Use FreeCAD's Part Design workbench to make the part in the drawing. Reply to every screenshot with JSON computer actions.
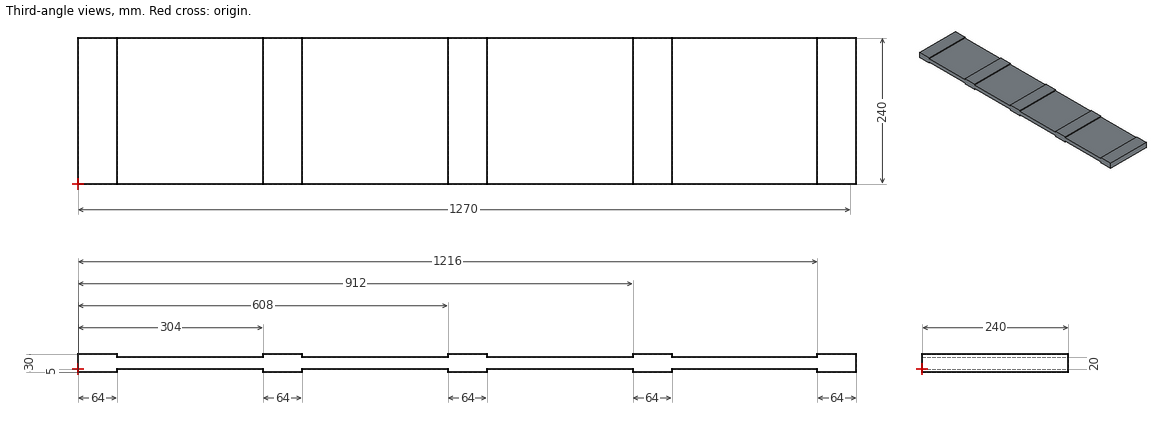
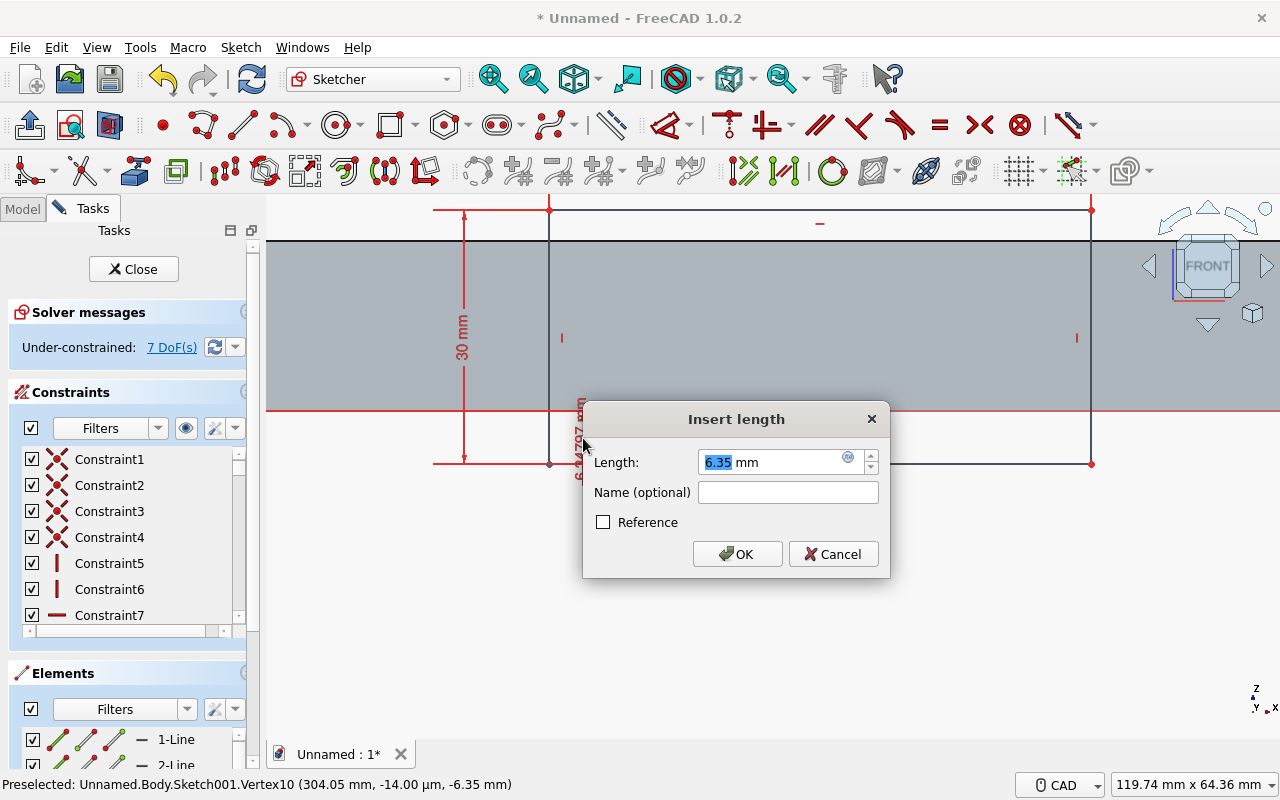
{"action": "type", "text": "5"}
{"action": "key", "text": "Return"}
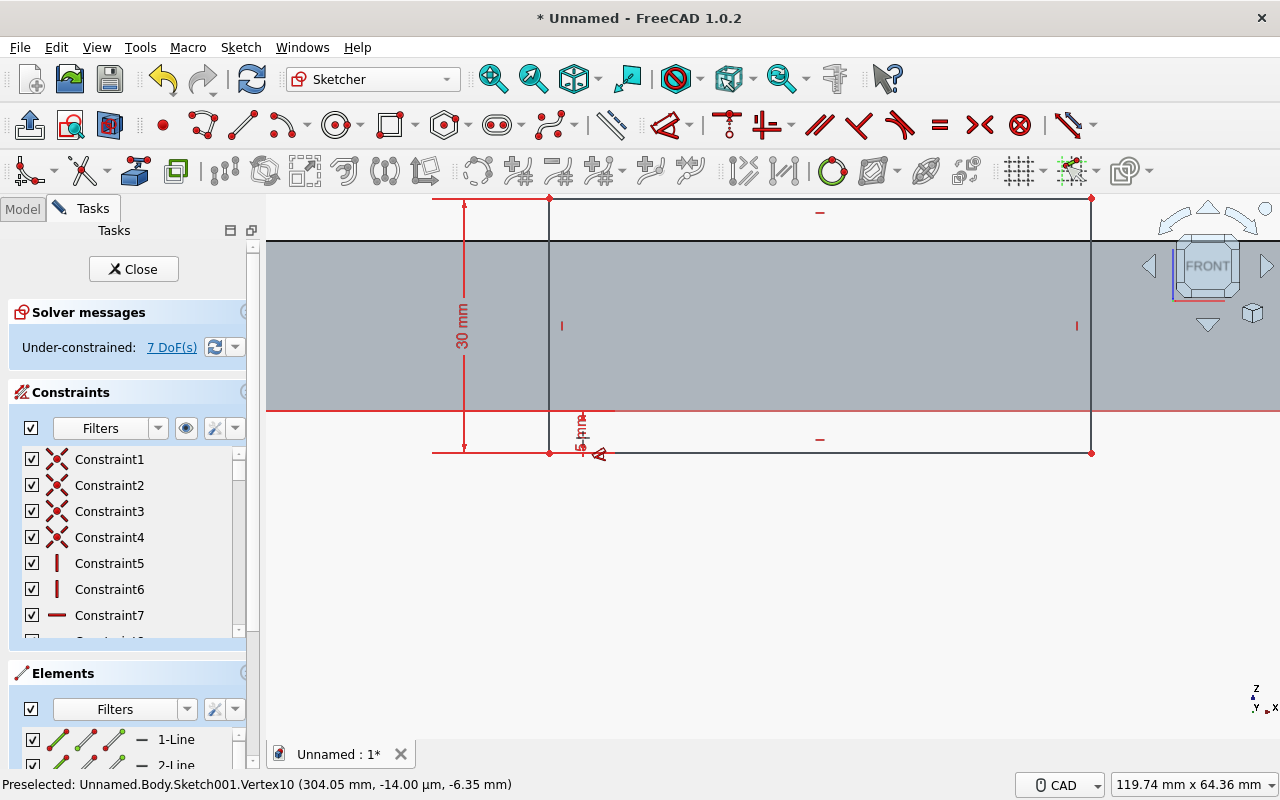
{"action": "scroll", "coordinate": [564, 474], "scroll_direction": "down", "scroll_amount": 15}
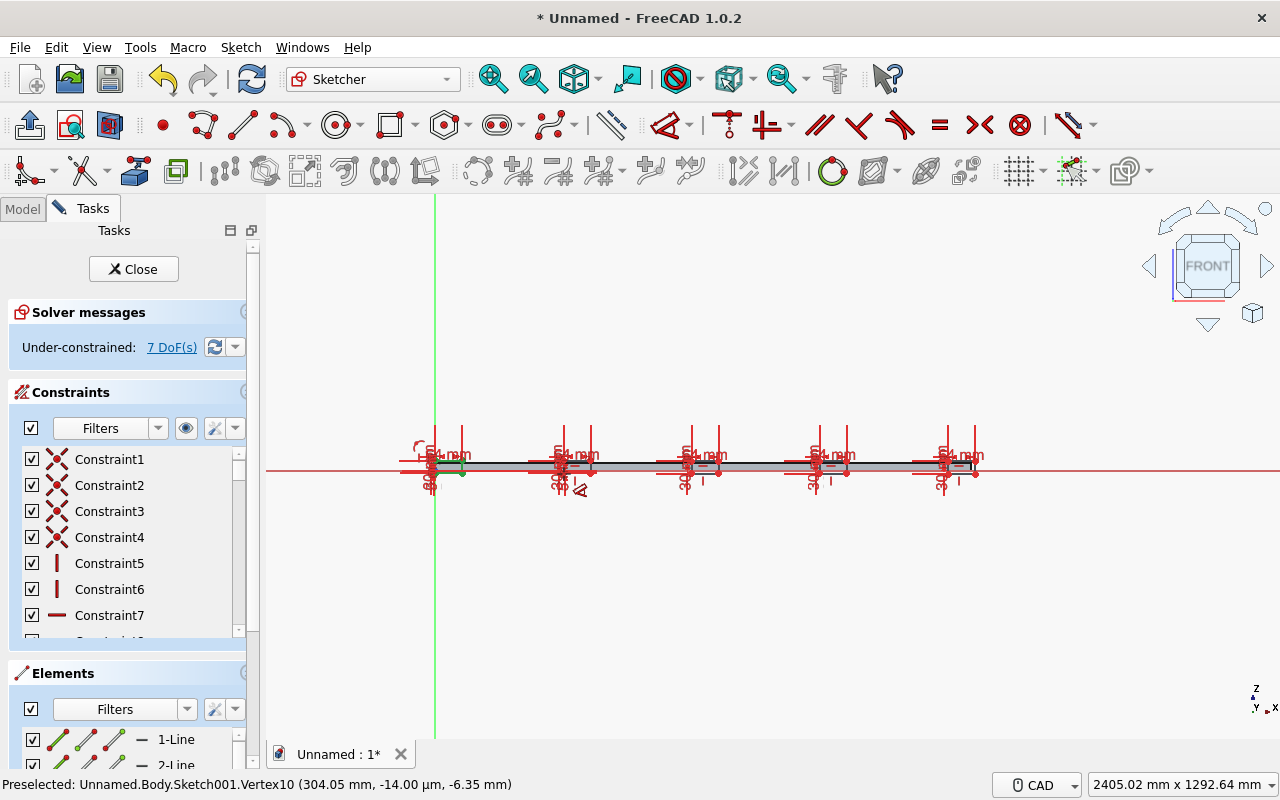
{"action": "scroll", "coordinate": [692, 474], "scroll_direction": "up", "scroll_amount": 15}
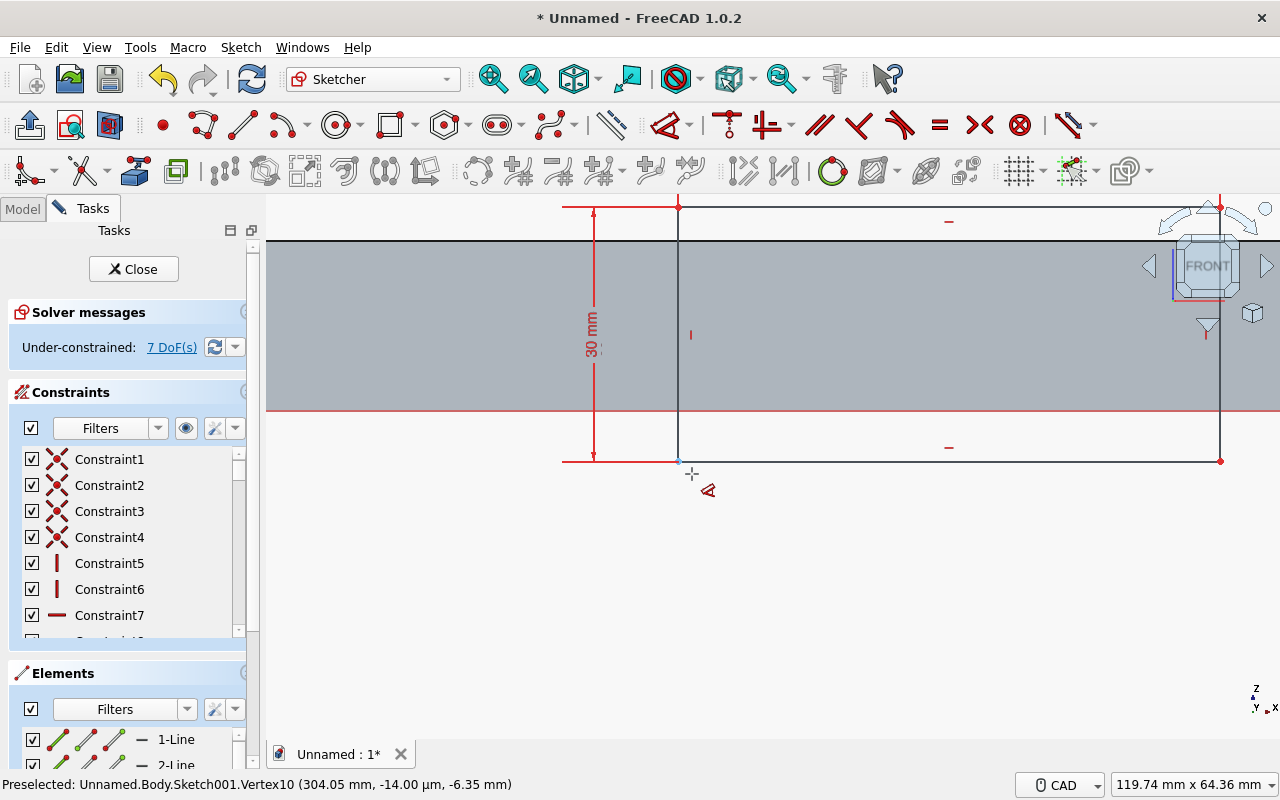
{"action": "left_click", "coordinate": [678, 462]}
{"action": "left_click", "coordinate": [712, 436]}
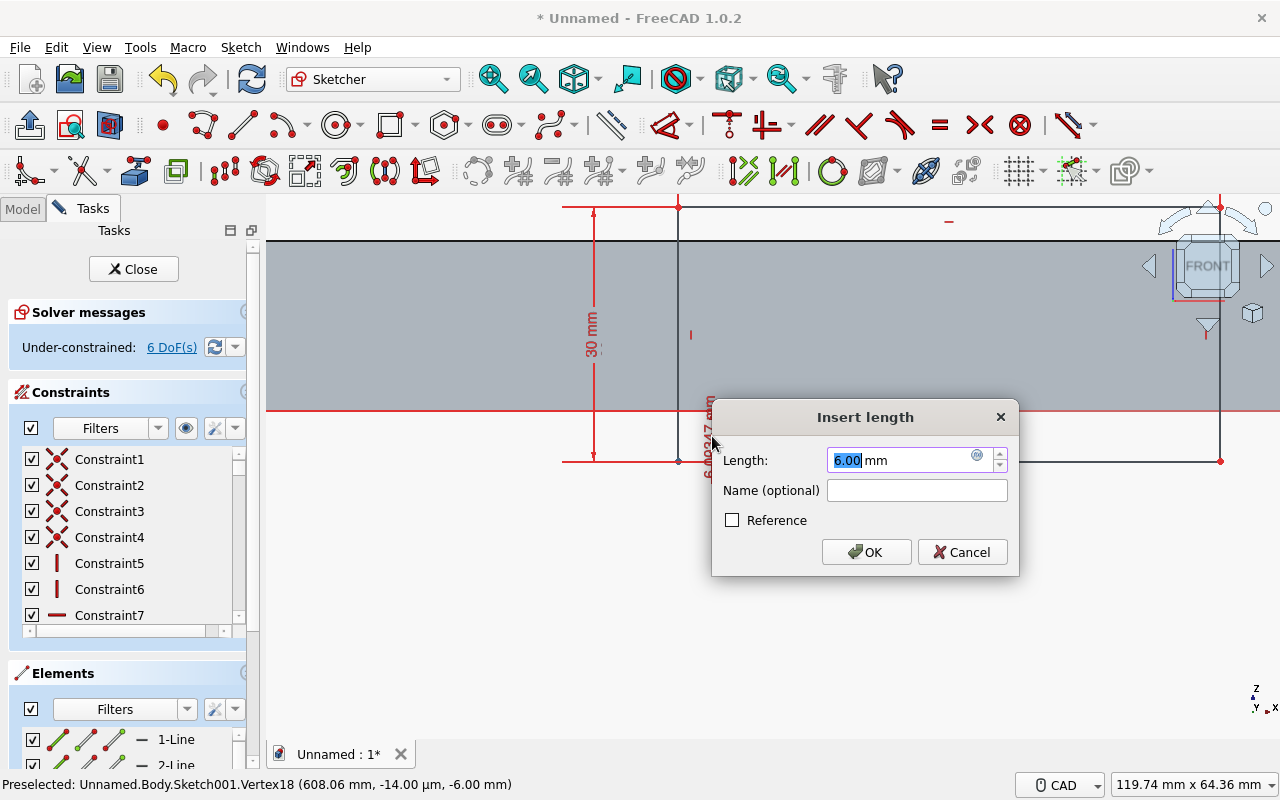
{"action": "type", "text": "5"}
{"action": "key", "text": "Return"}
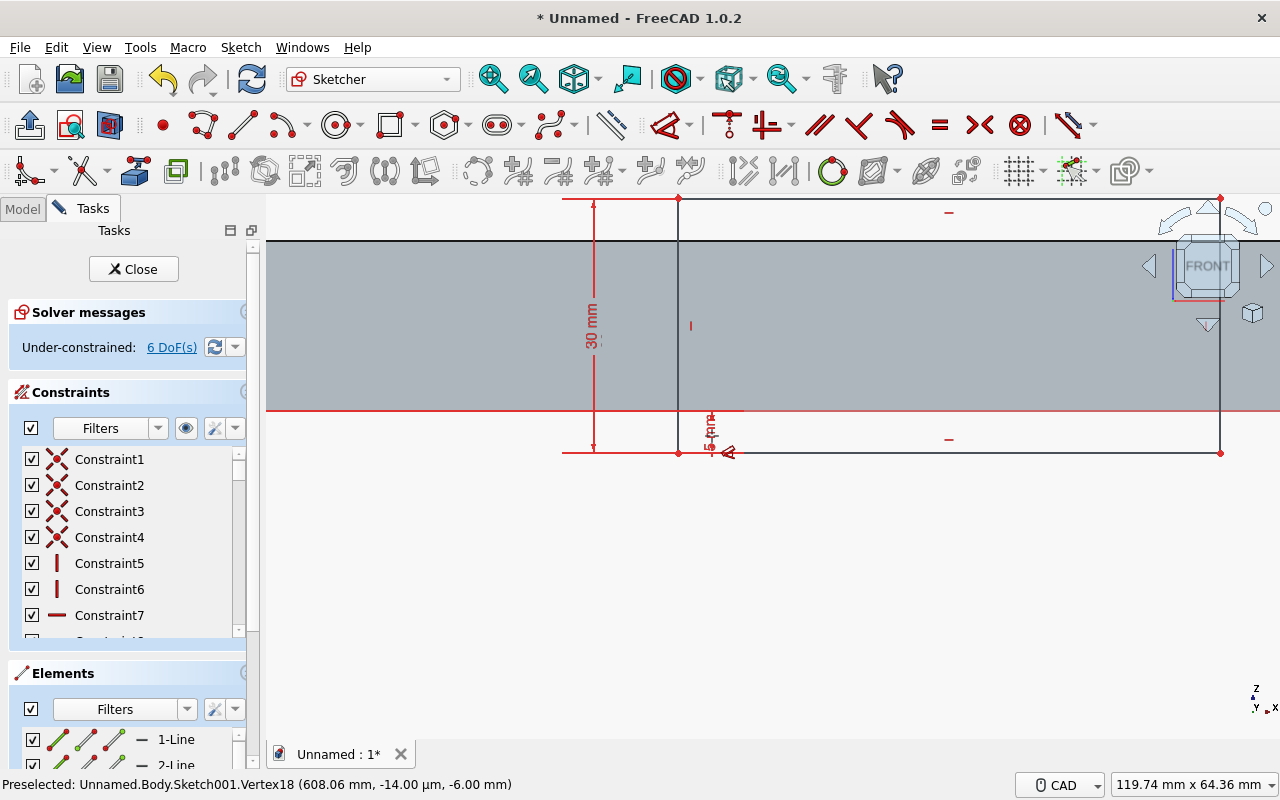
{"action": "scroll", "coordinate": [692, 474], "scroll_direction": "down", "scroll_amount": 15}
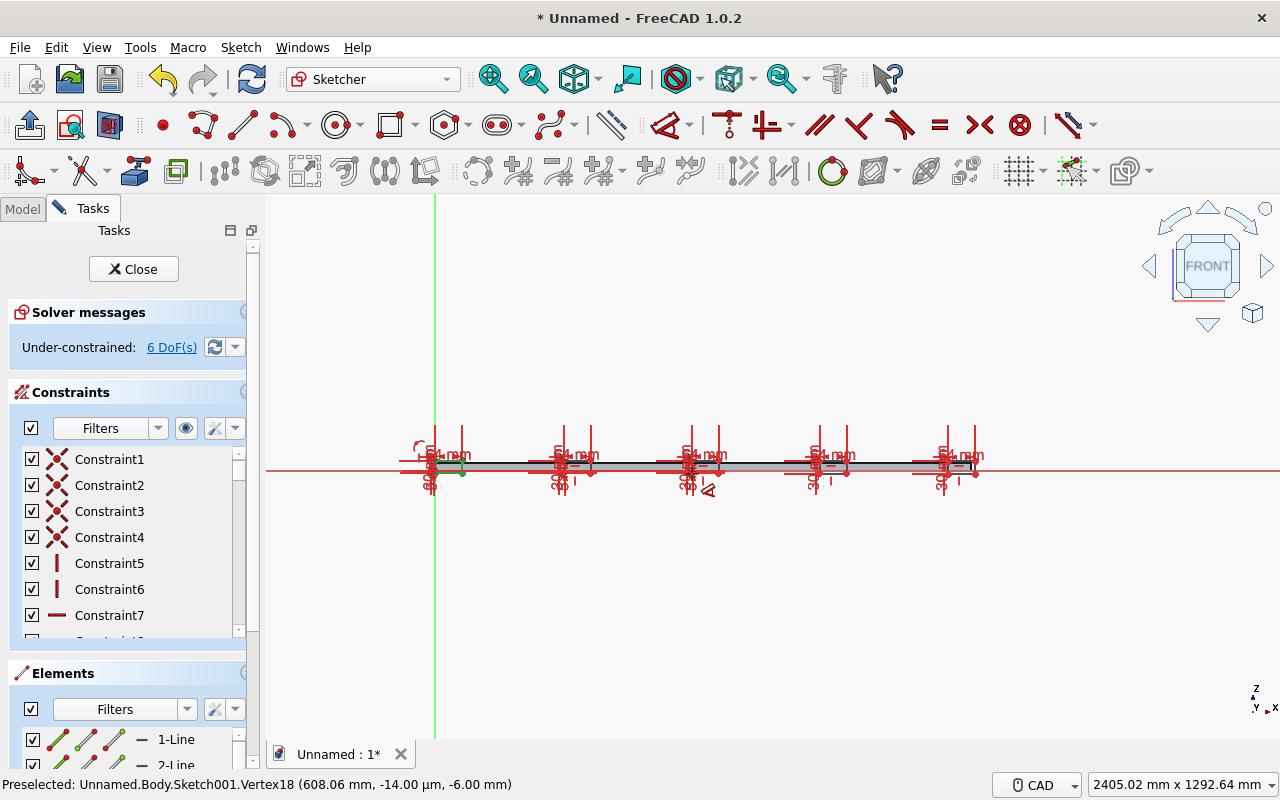
{"action": "scroll", "coordinate": [820, 474], "scroll_direction": "up", "scroll_amount": 15}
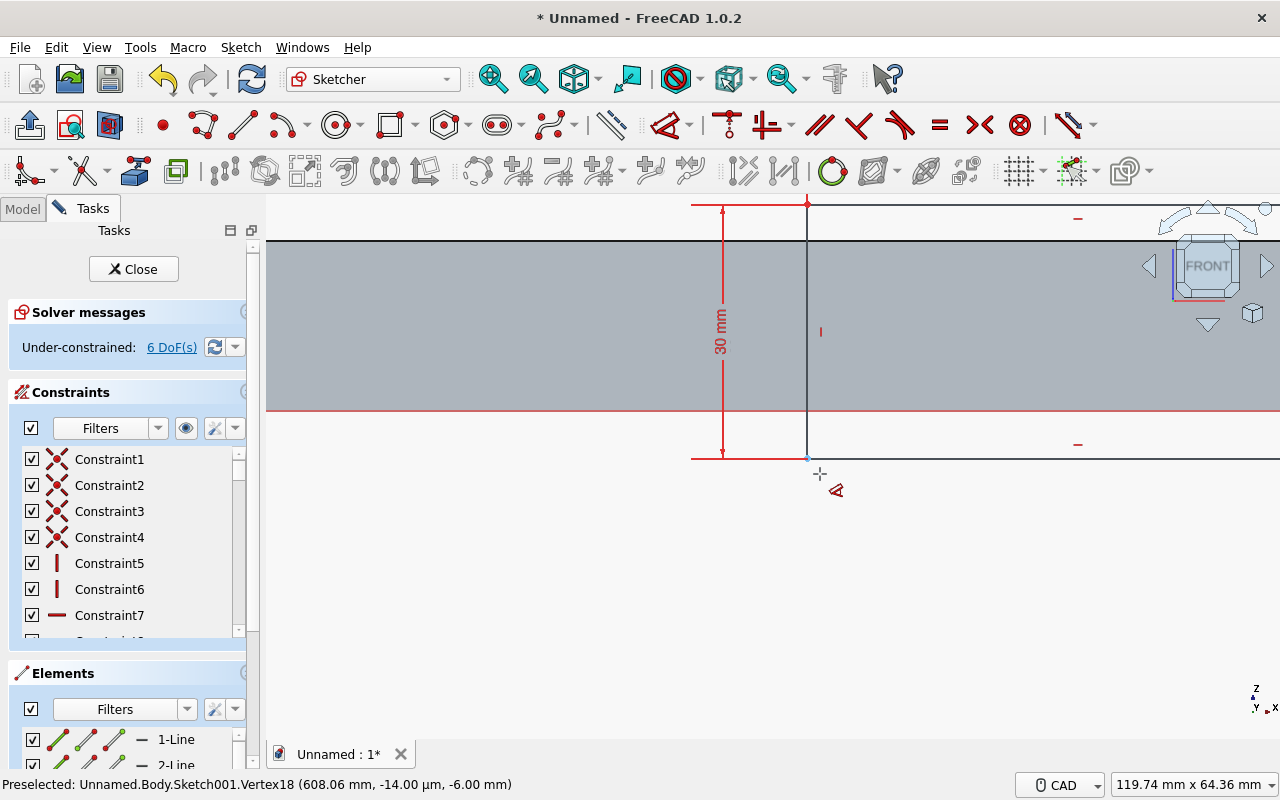
{"action": "left_click", "coordinate": [807, 459]}
{"action": "left_click", "coordinate": [841, 435]}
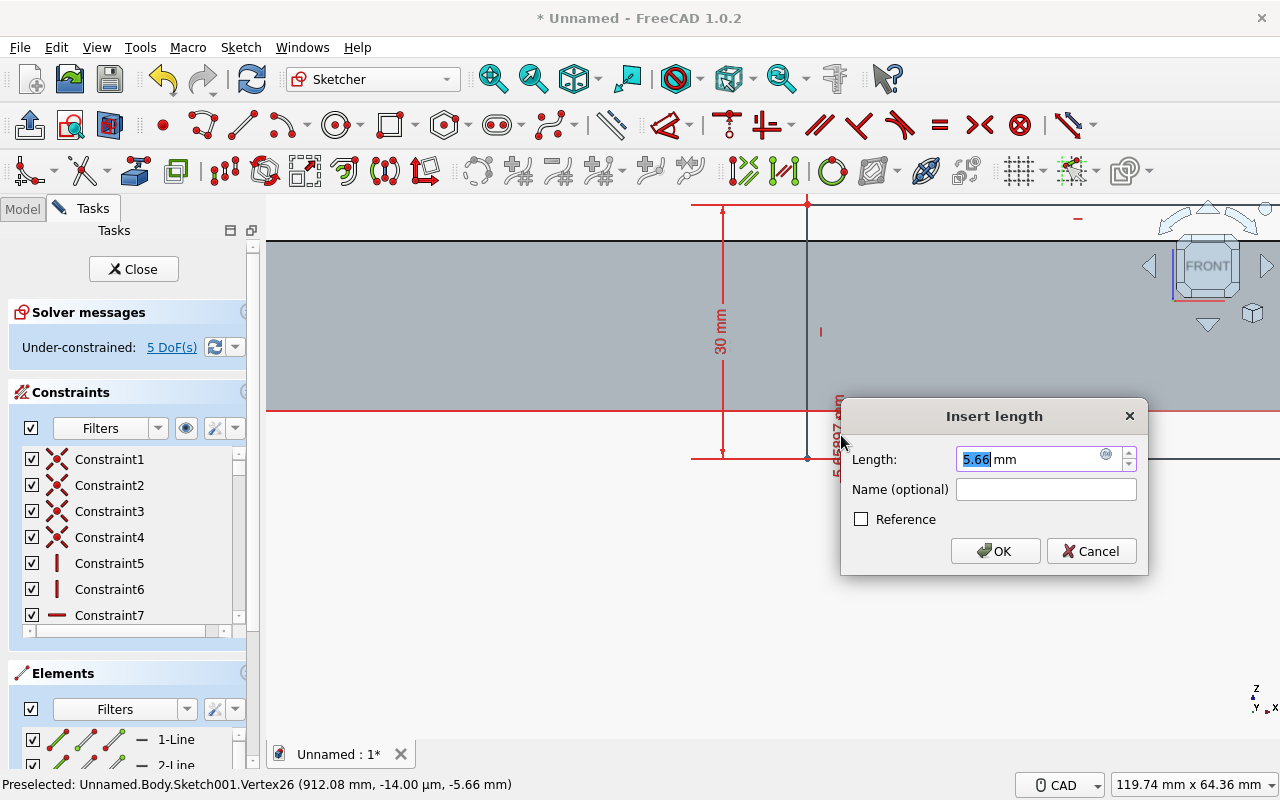
{"action": "type", "text": "5"}
{"action": "key", "text": "Return"}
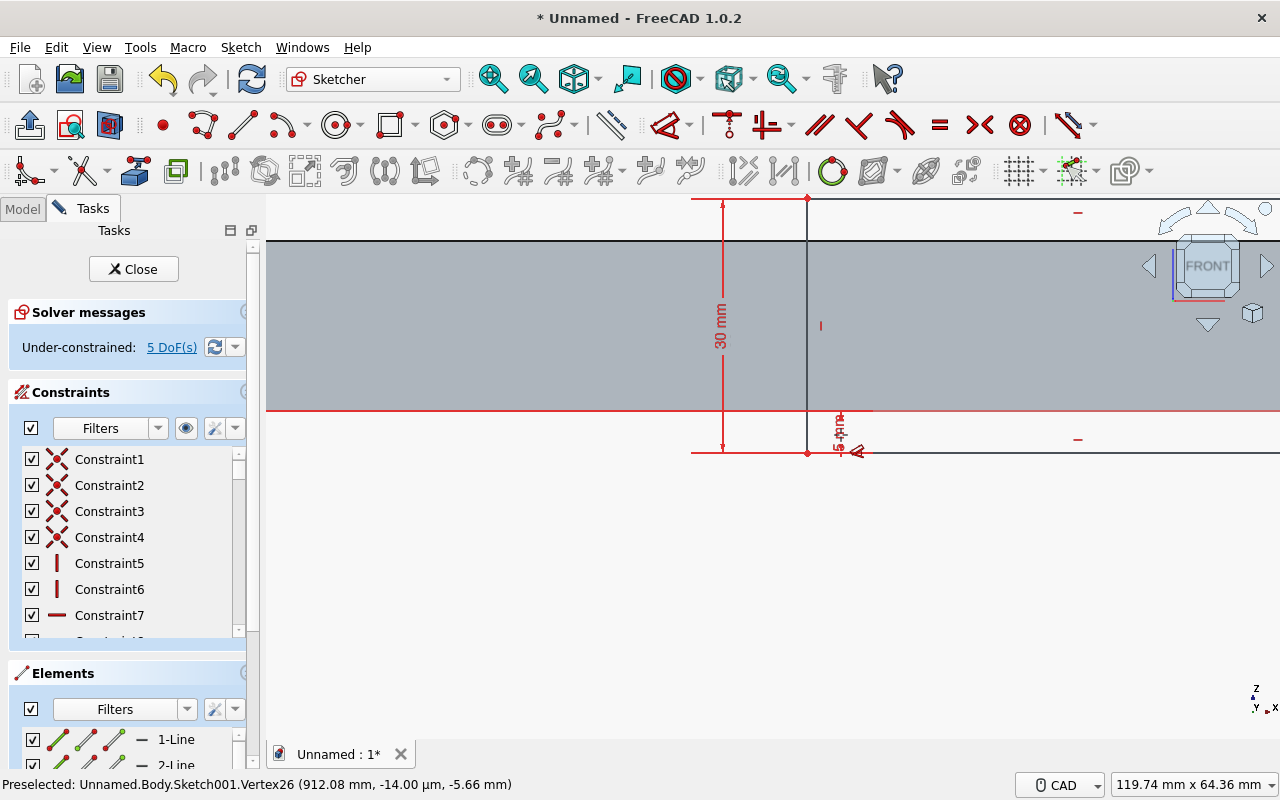
{"action": "scroll", "coordinate": [820, 474], "scroll_direction": "down", "scroll_amount": 15}